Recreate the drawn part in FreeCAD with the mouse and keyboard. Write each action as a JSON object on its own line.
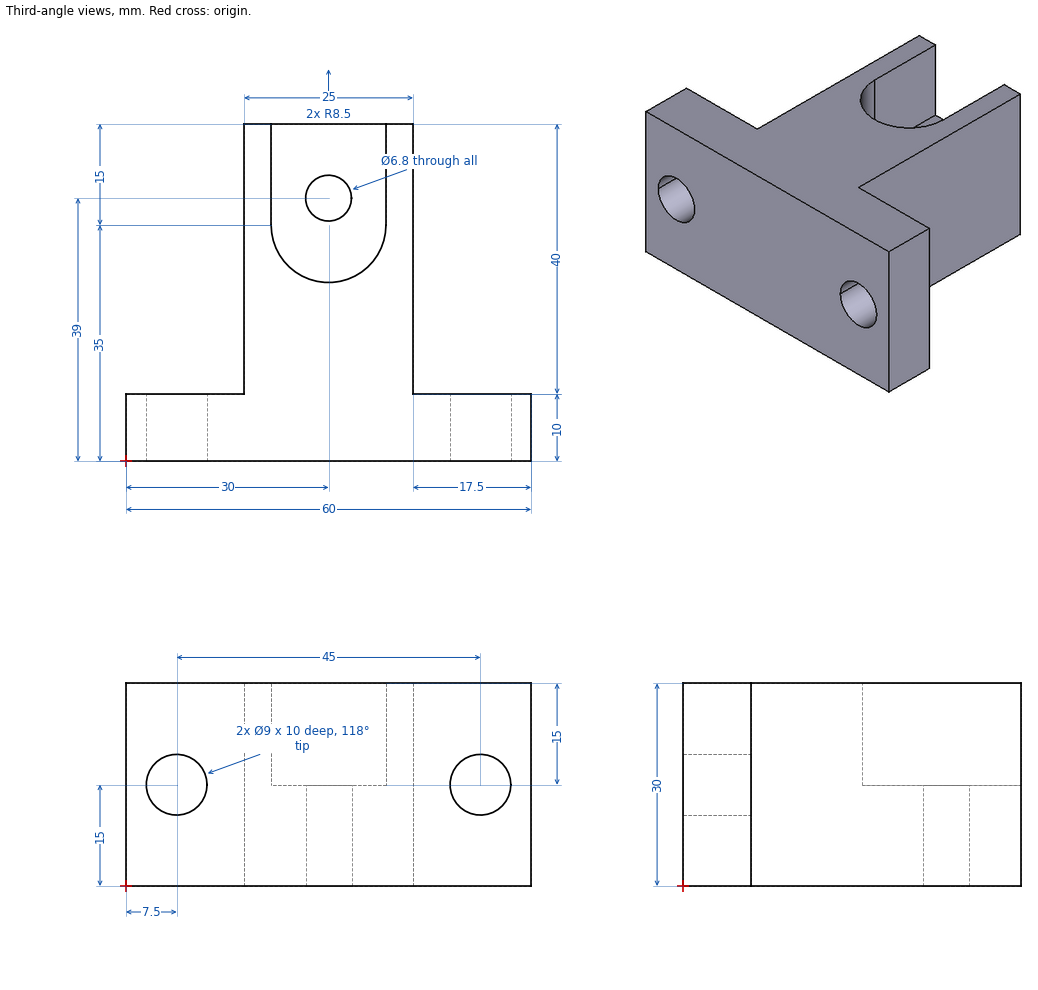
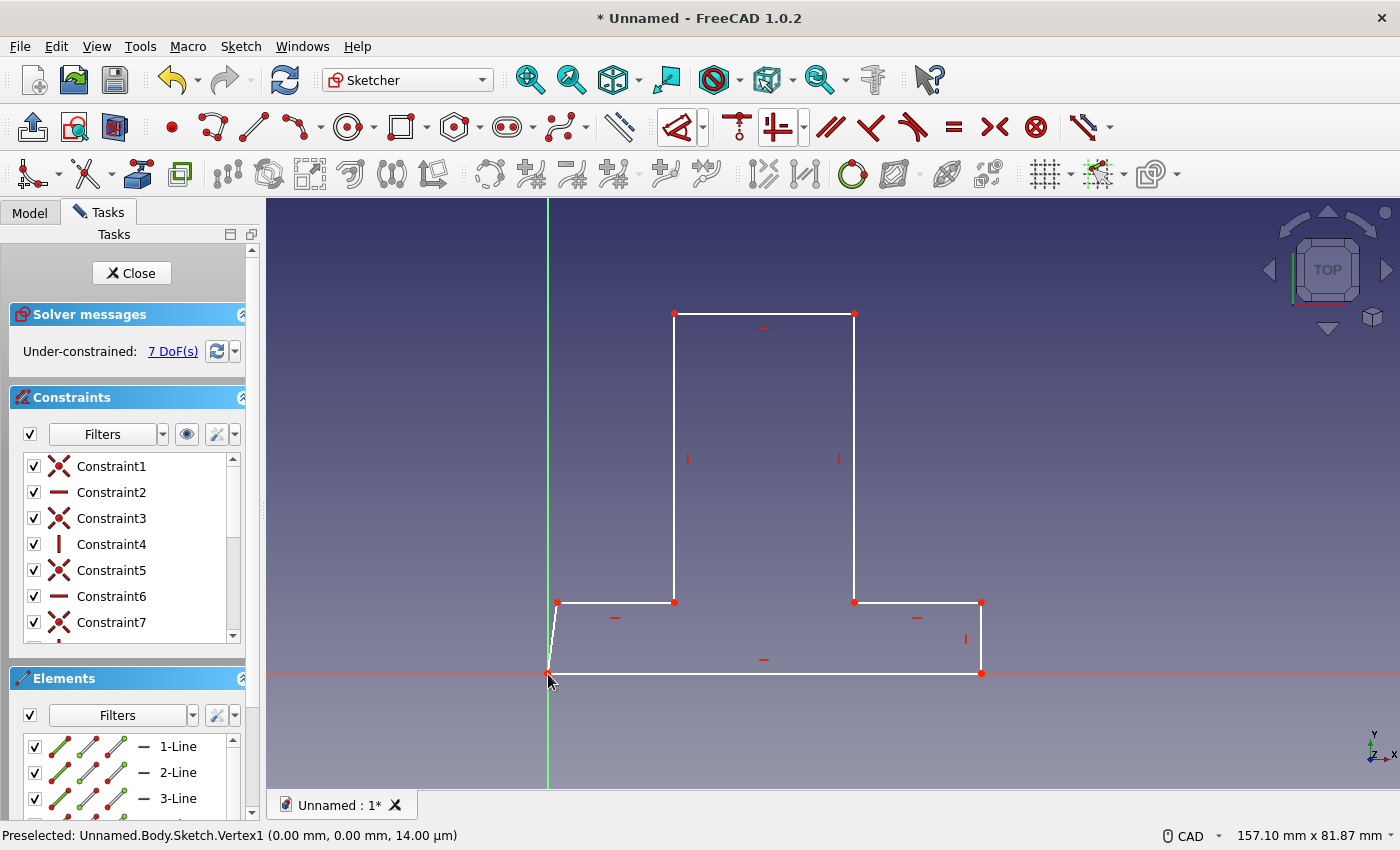
{"action": "left_click", "coordinate": [550, 653]}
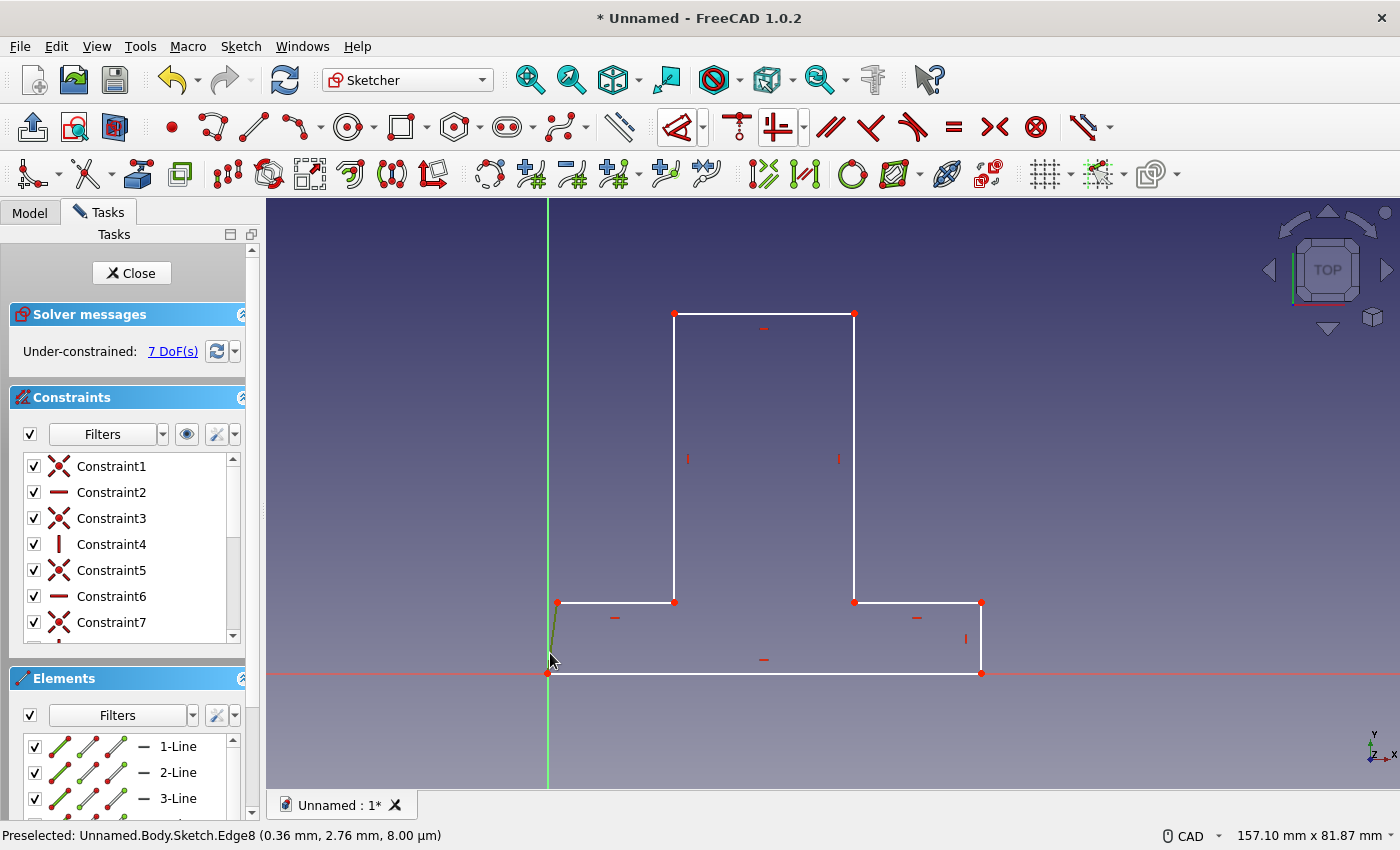
{"action": "key", "text": "v"}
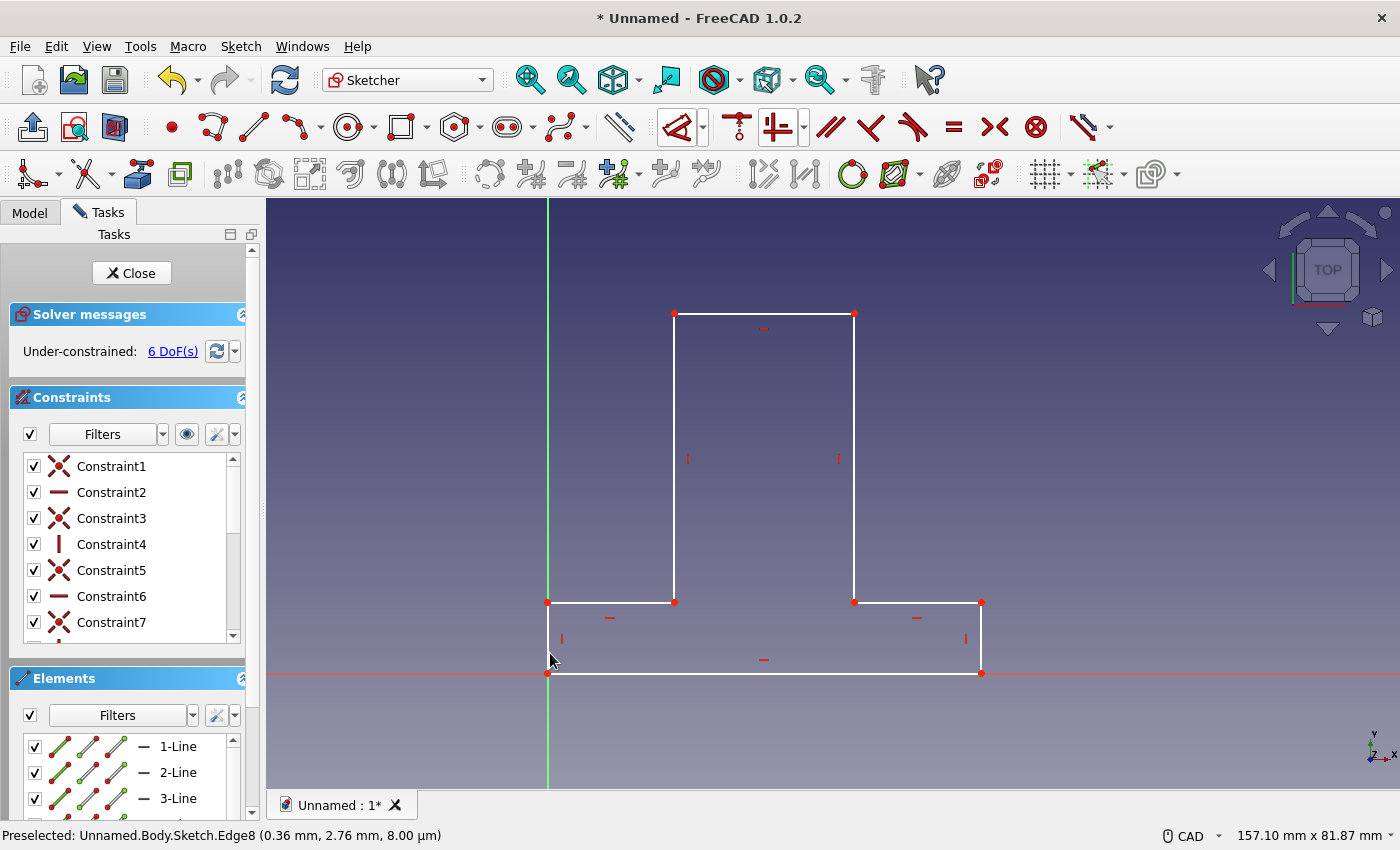
{"action": "left_click", "coordinate": [676, 128]}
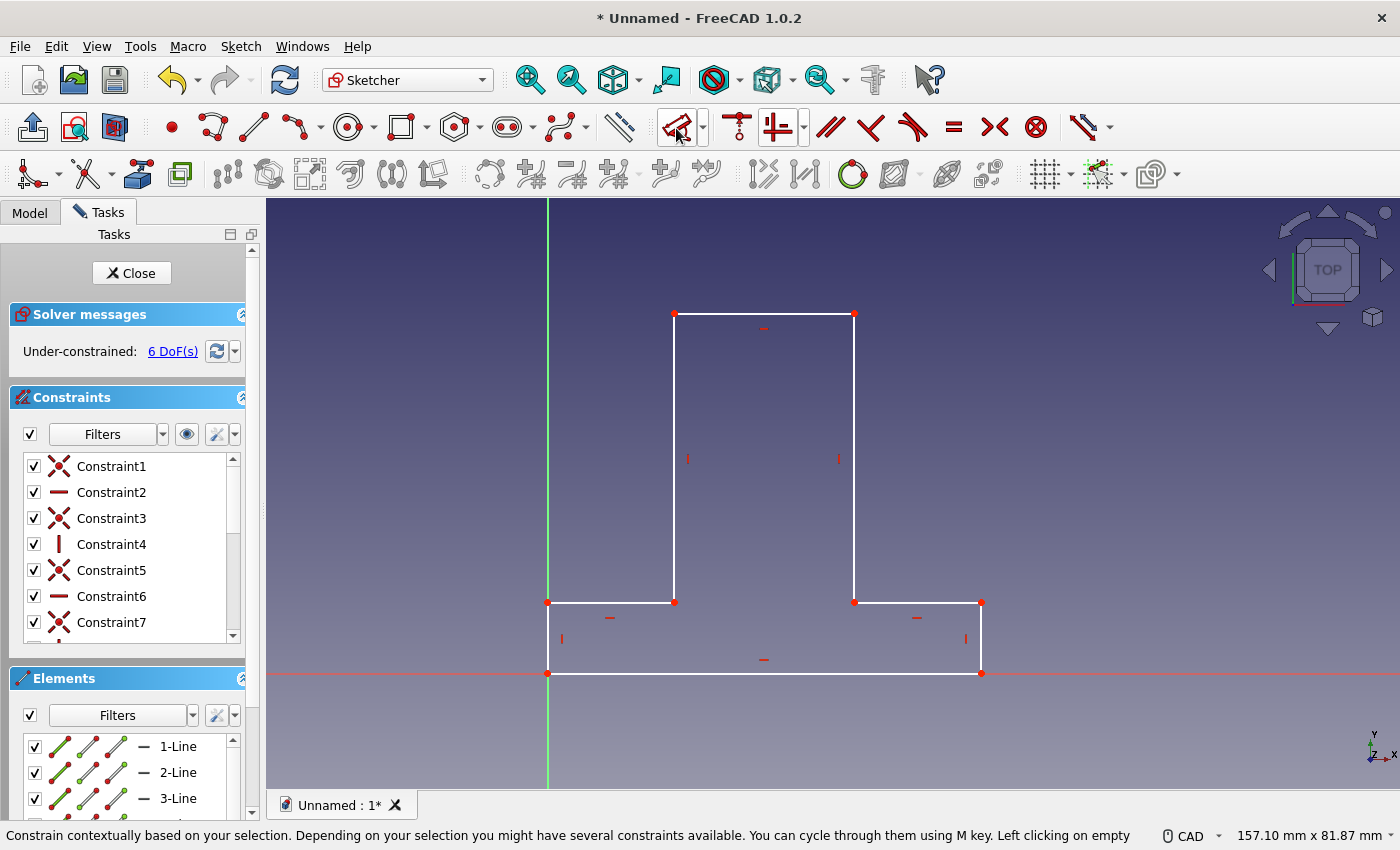
{"action": "left_click", "coordinate": [678, 674]}
{"action": "left_click", "coordinate": [764, 708]}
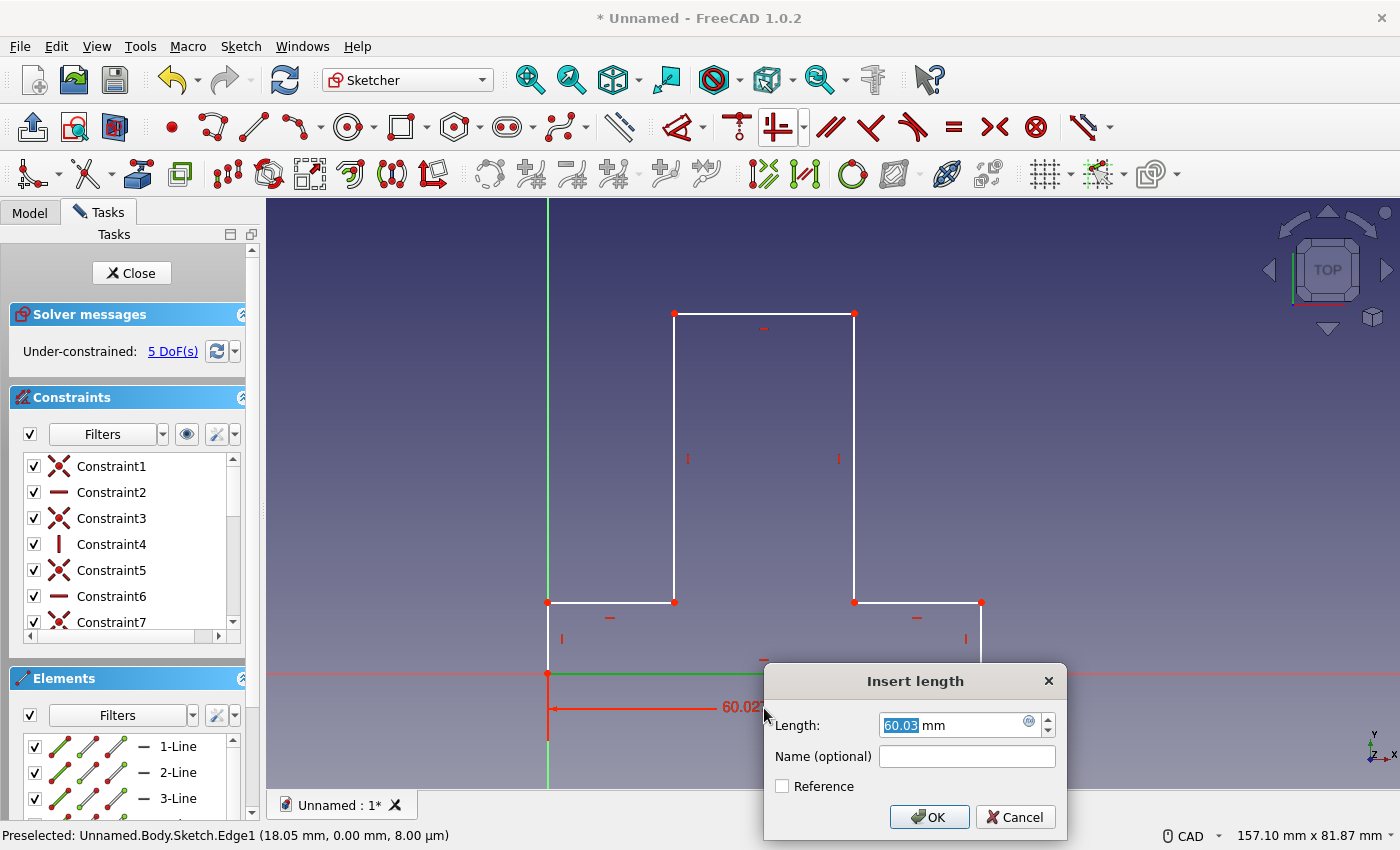
{"action": "type", "text": "60"}
{"action": "key", "text": "Return"}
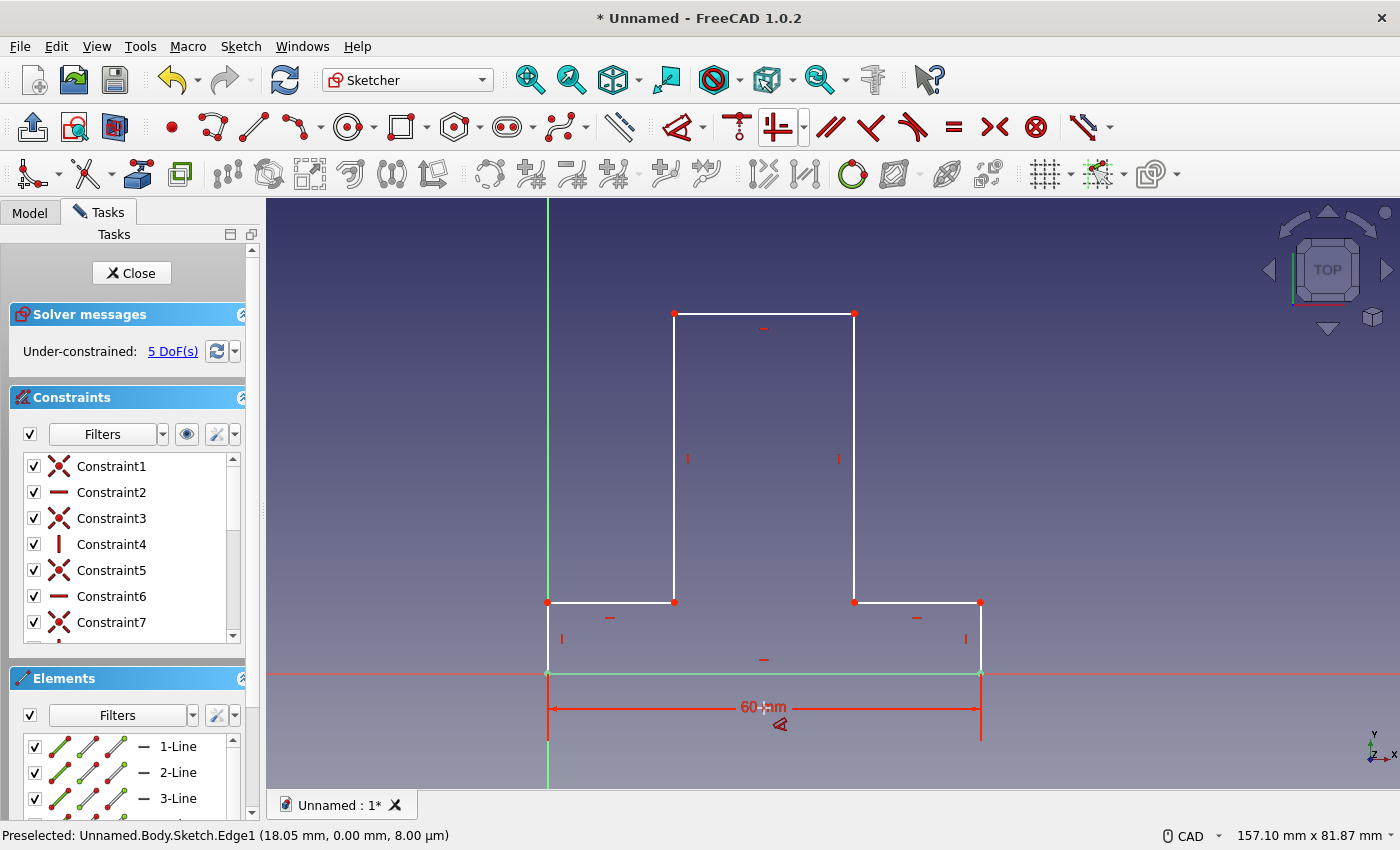
{"action": "left_click", "coordinate": [981, 653]}
{"action": "left_click", "coordinate": [1015, 638]}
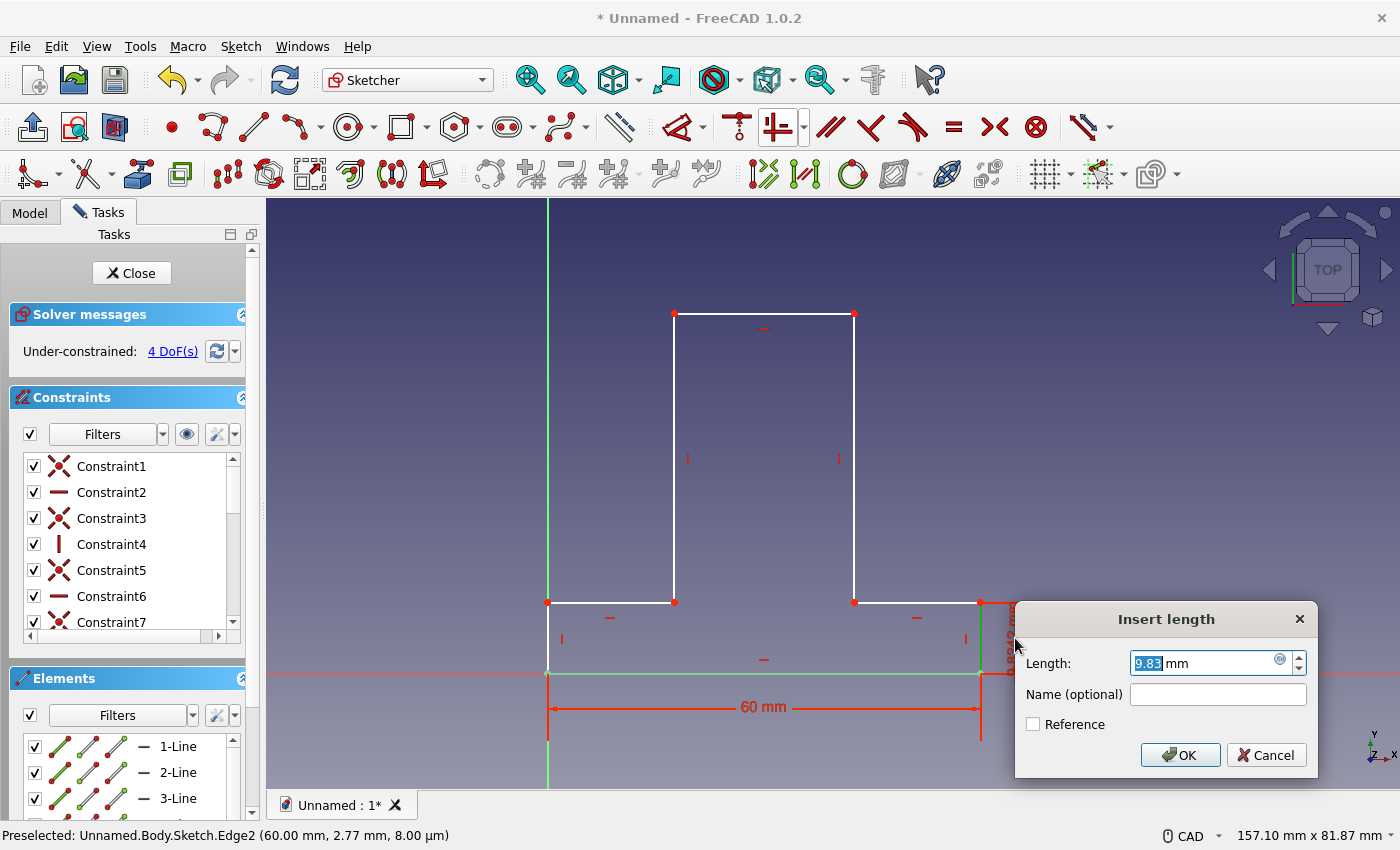
{"action": "type", "text": "10"}
{"action": "key", "text": "Return"}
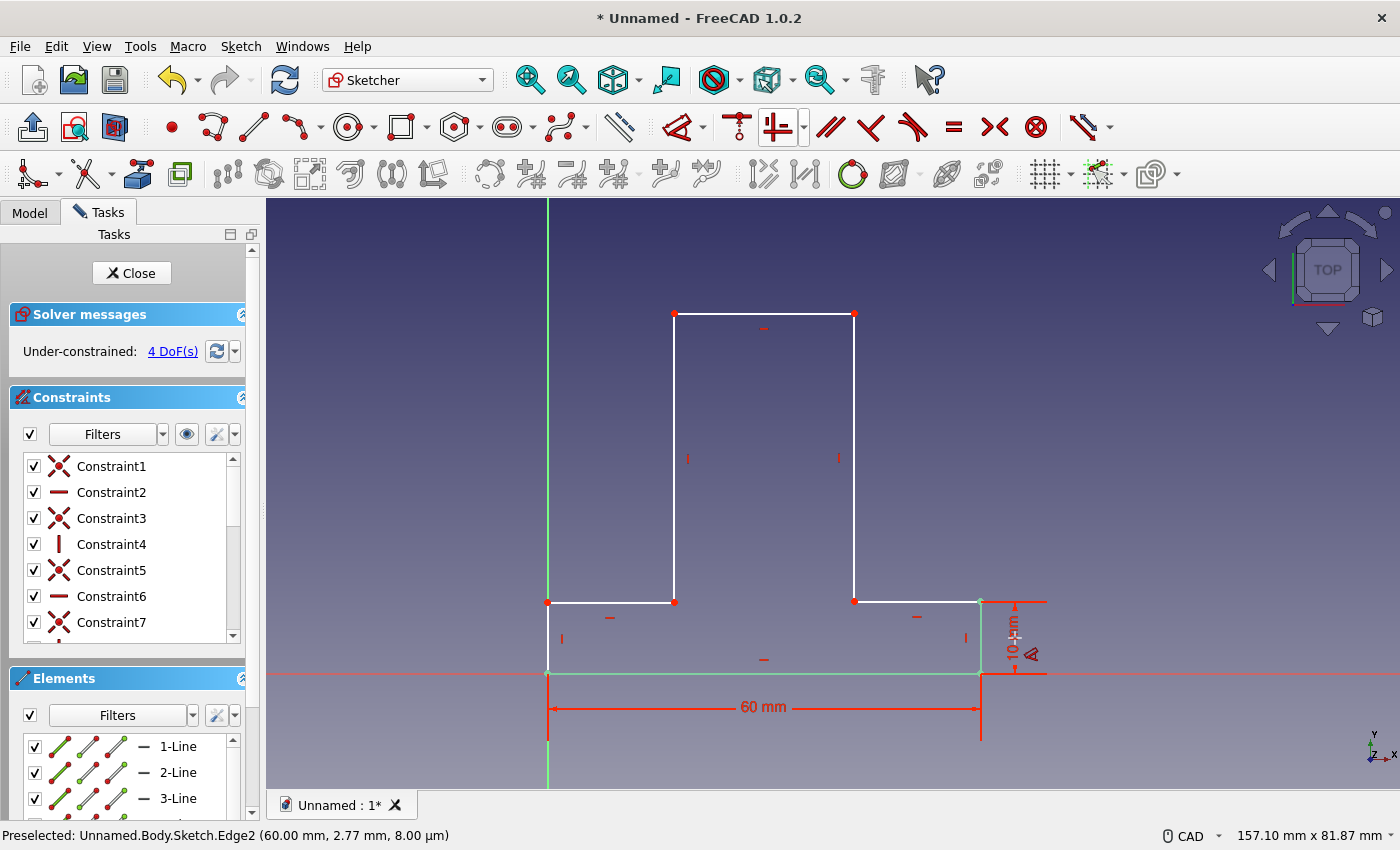
{"action": "left_click", "coordinate": [854, 515]}
{"action": "left_click", "coordinate": [888, 458]}